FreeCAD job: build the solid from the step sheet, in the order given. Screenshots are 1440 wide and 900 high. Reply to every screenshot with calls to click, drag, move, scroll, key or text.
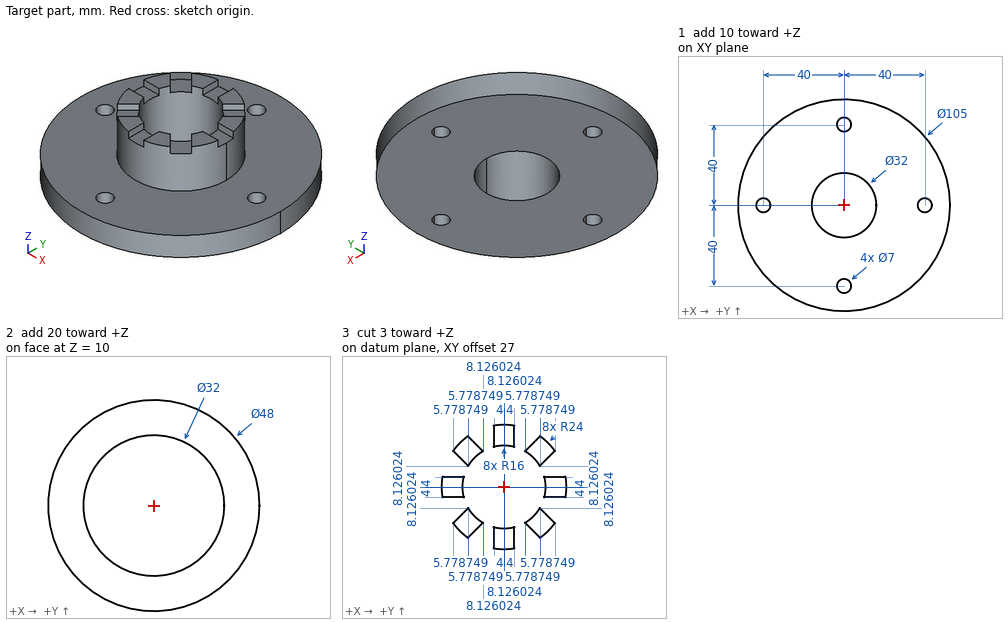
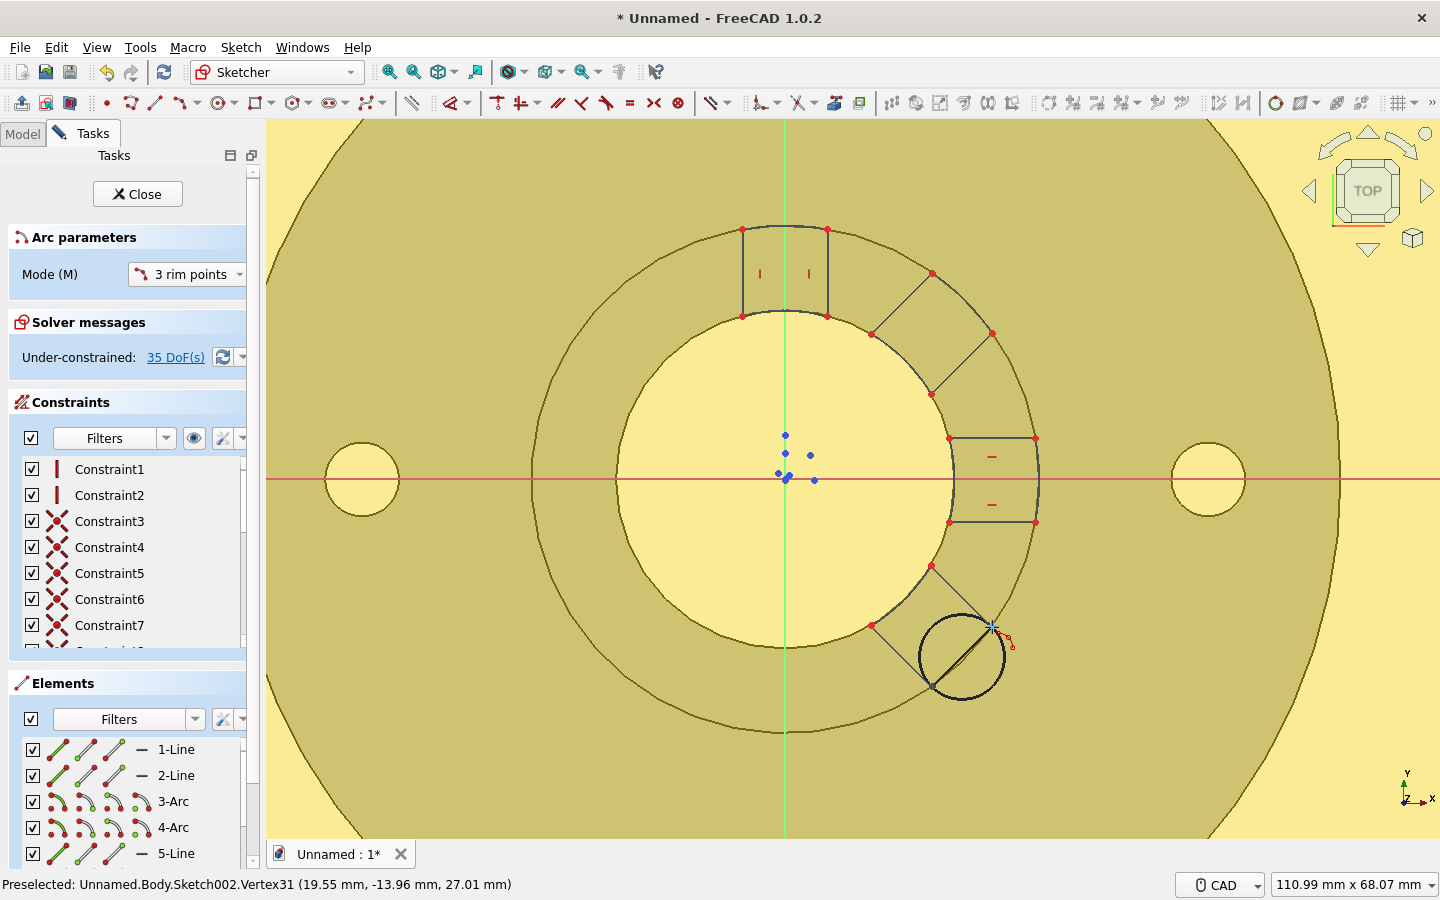
scroll(965, 659, up, 8)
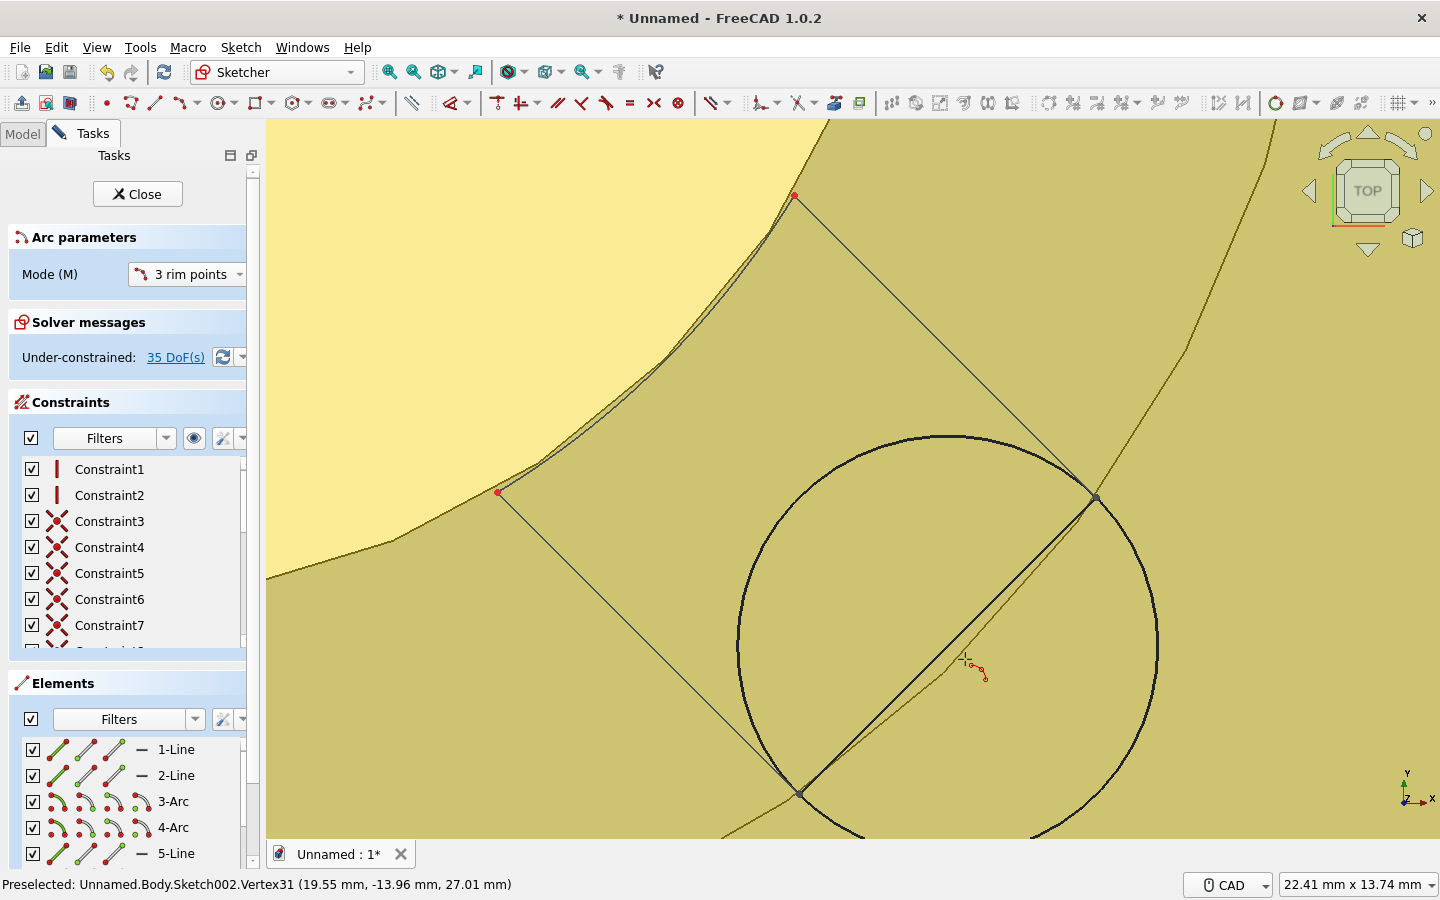
click(961, 655)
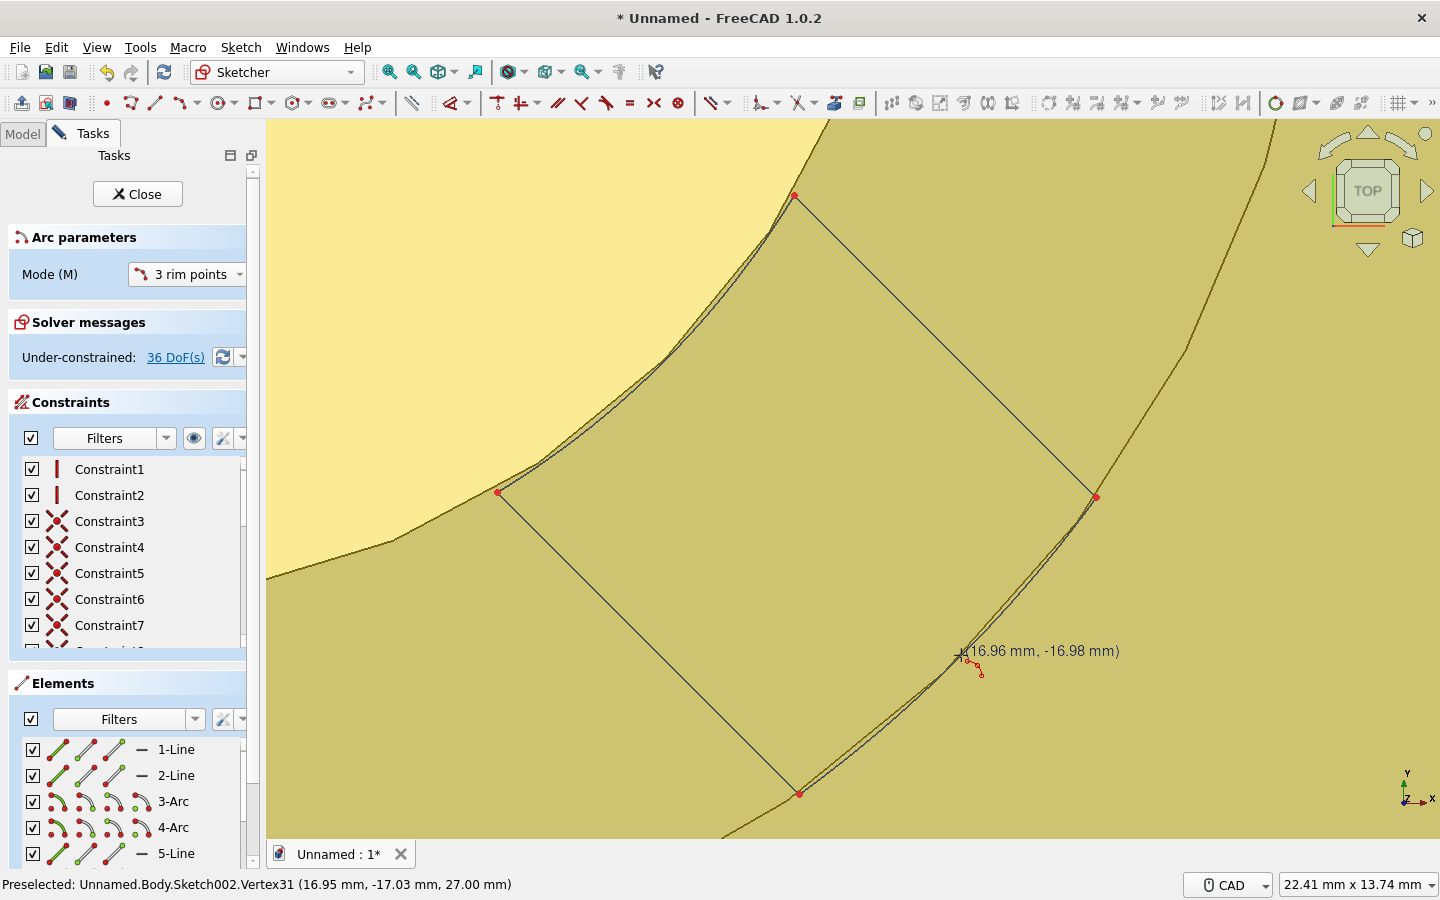
click(156, 104)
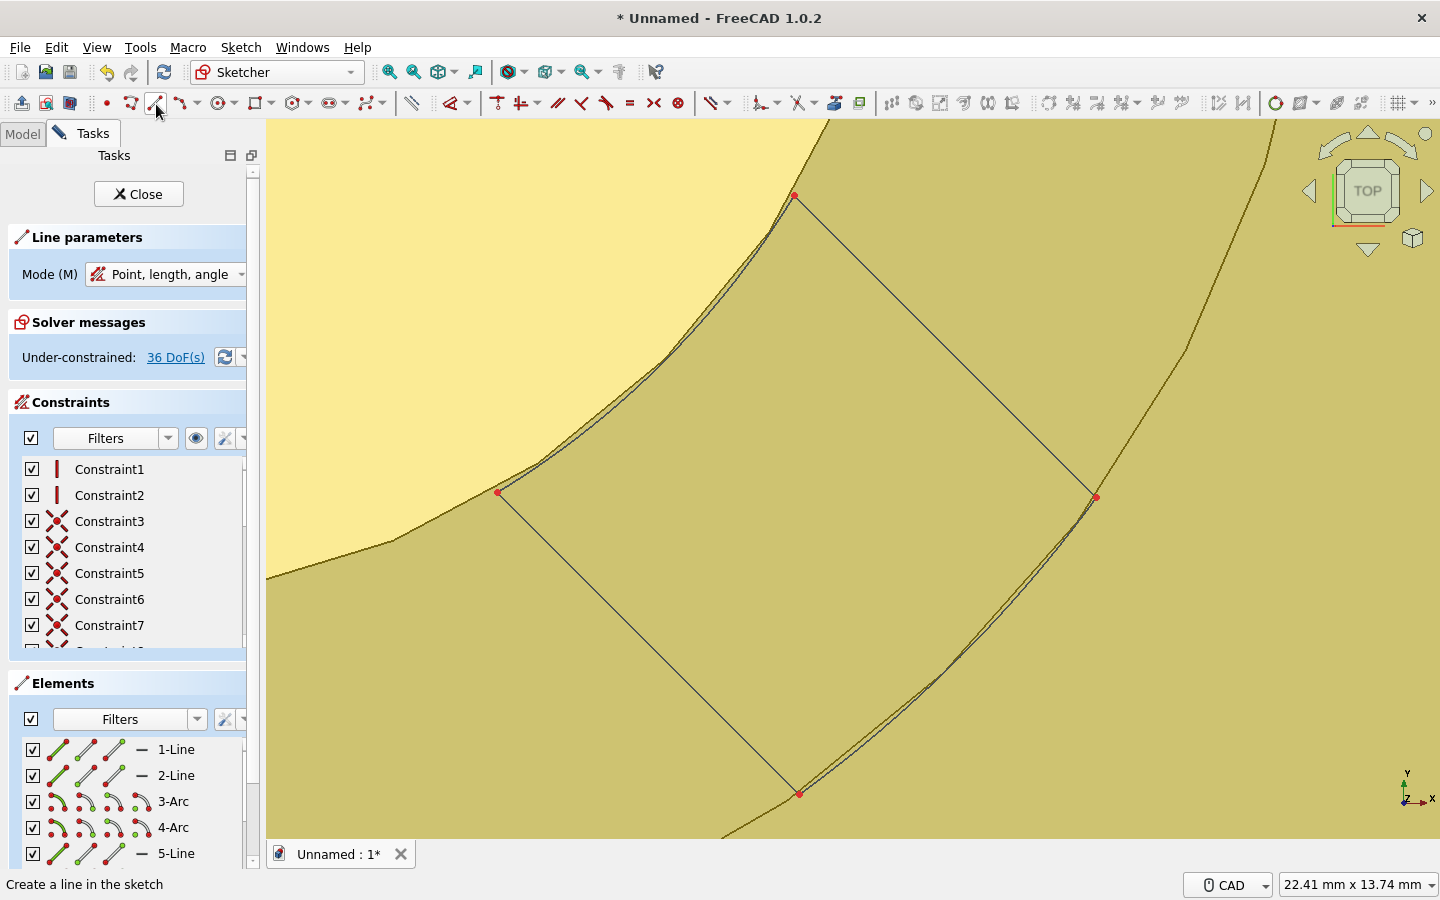
scroll(965, 659, down, 8)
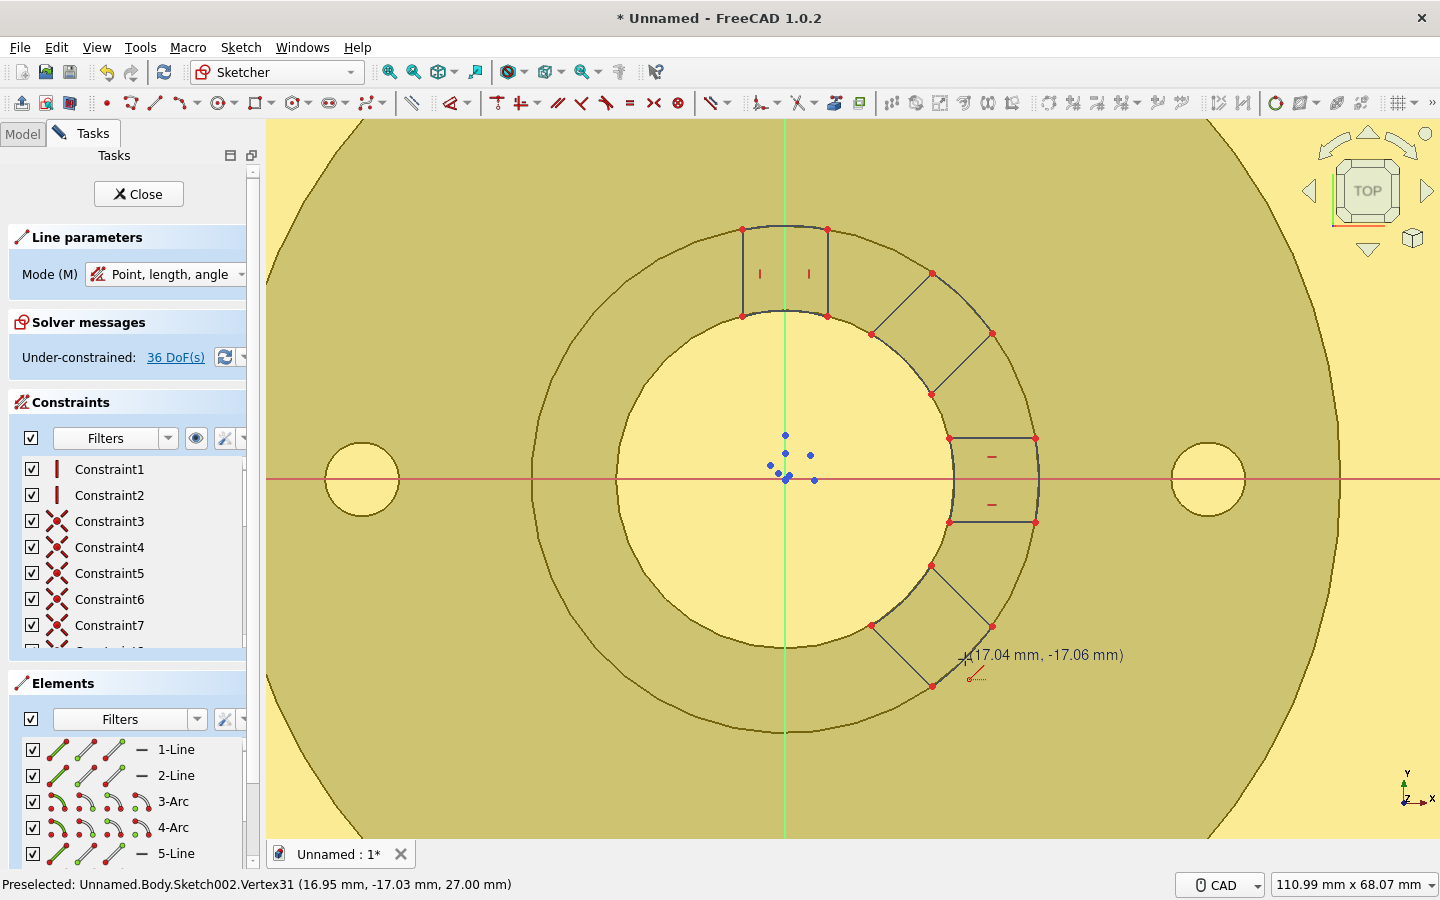
click(828, 730)
click(828, 643)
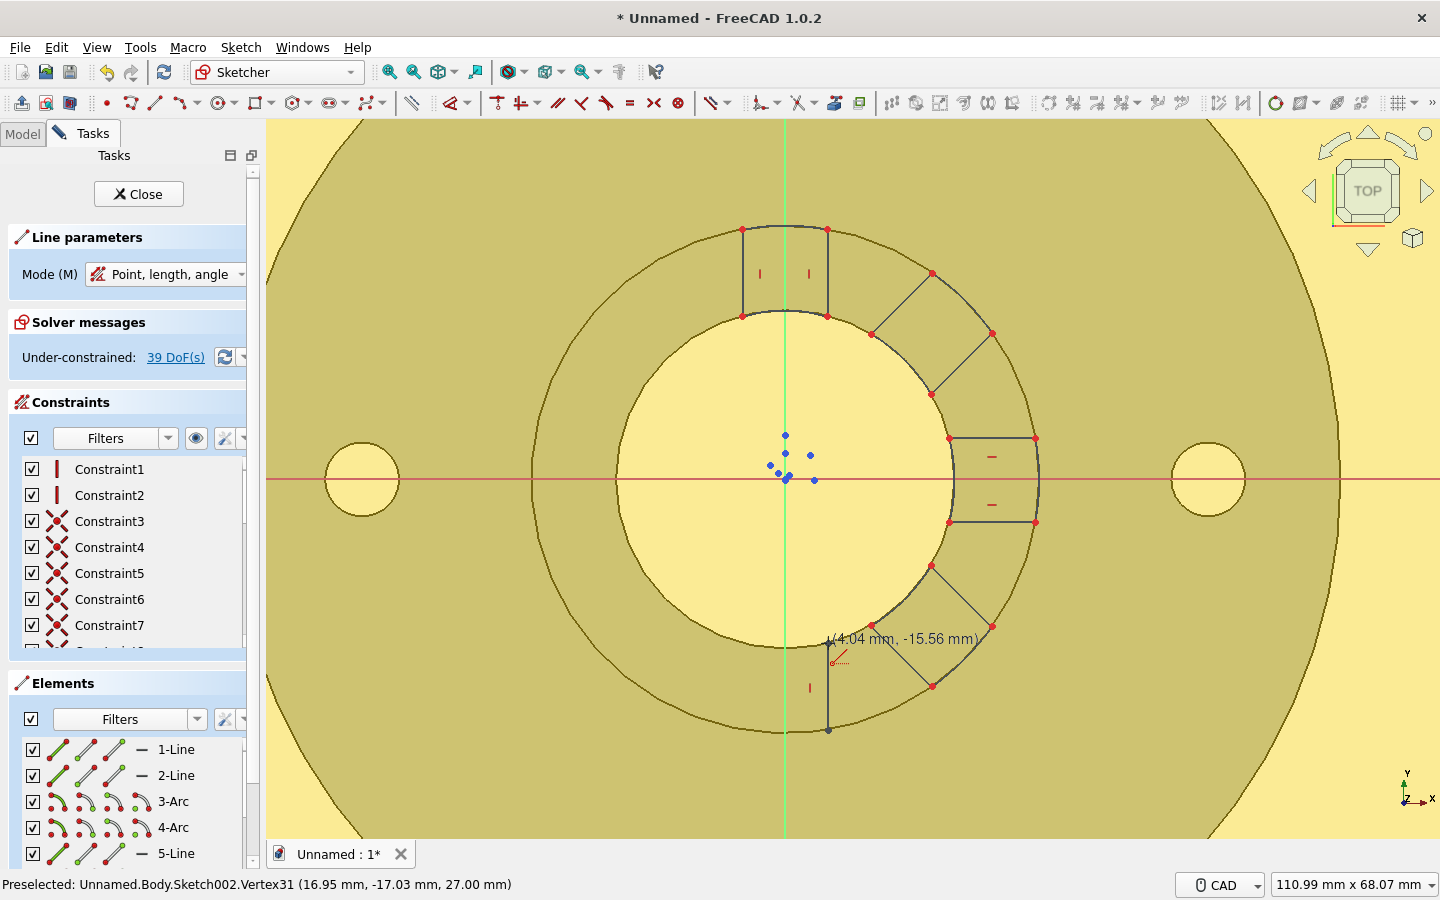
click(743, 643)
click(743, 730)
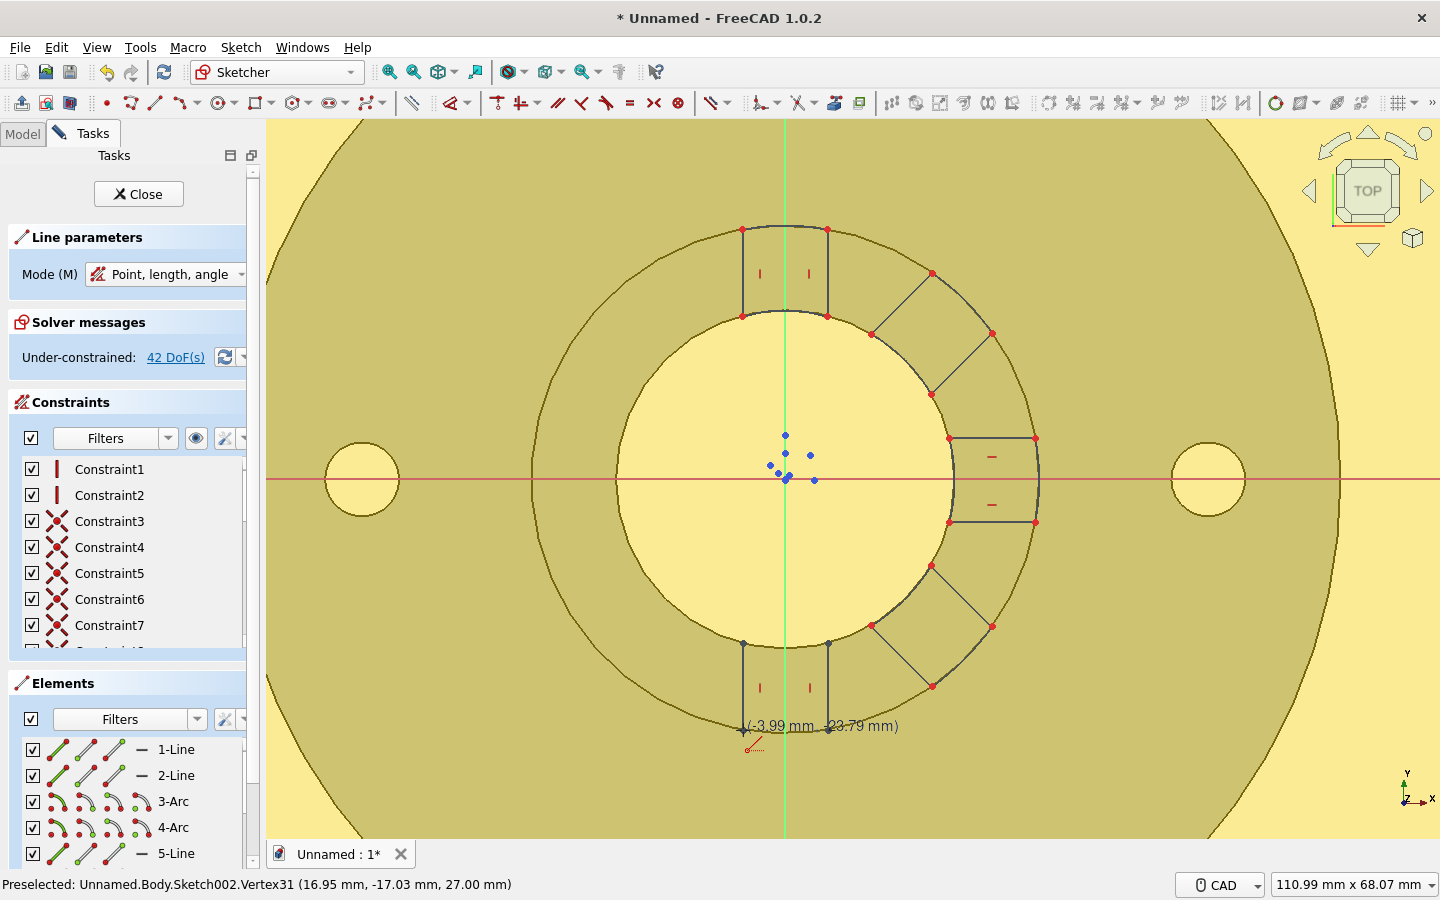
click(180, 104)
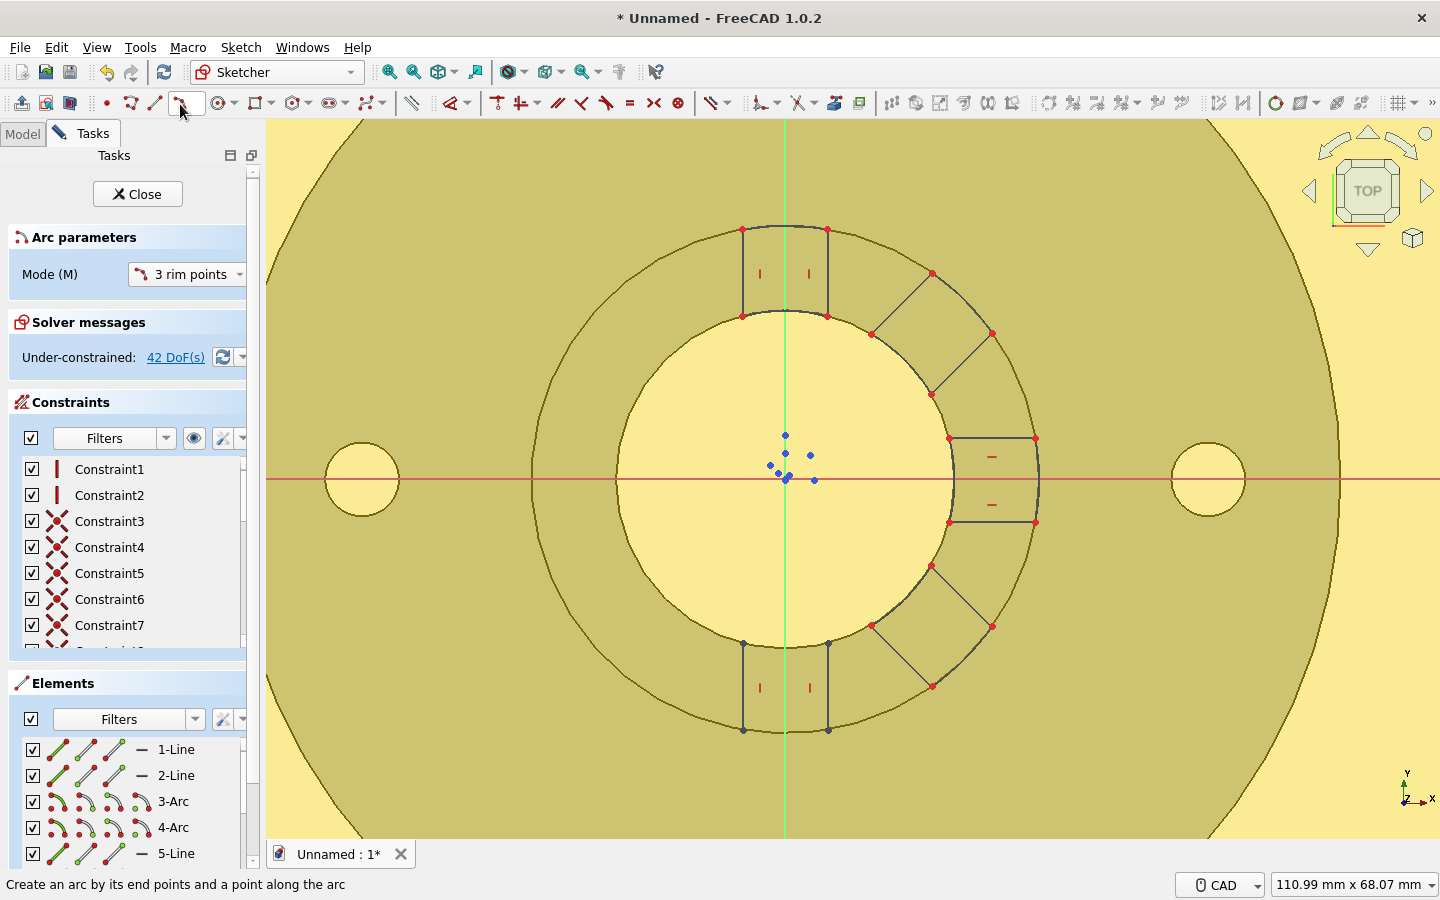
click(828, 644)
click(743, 644)